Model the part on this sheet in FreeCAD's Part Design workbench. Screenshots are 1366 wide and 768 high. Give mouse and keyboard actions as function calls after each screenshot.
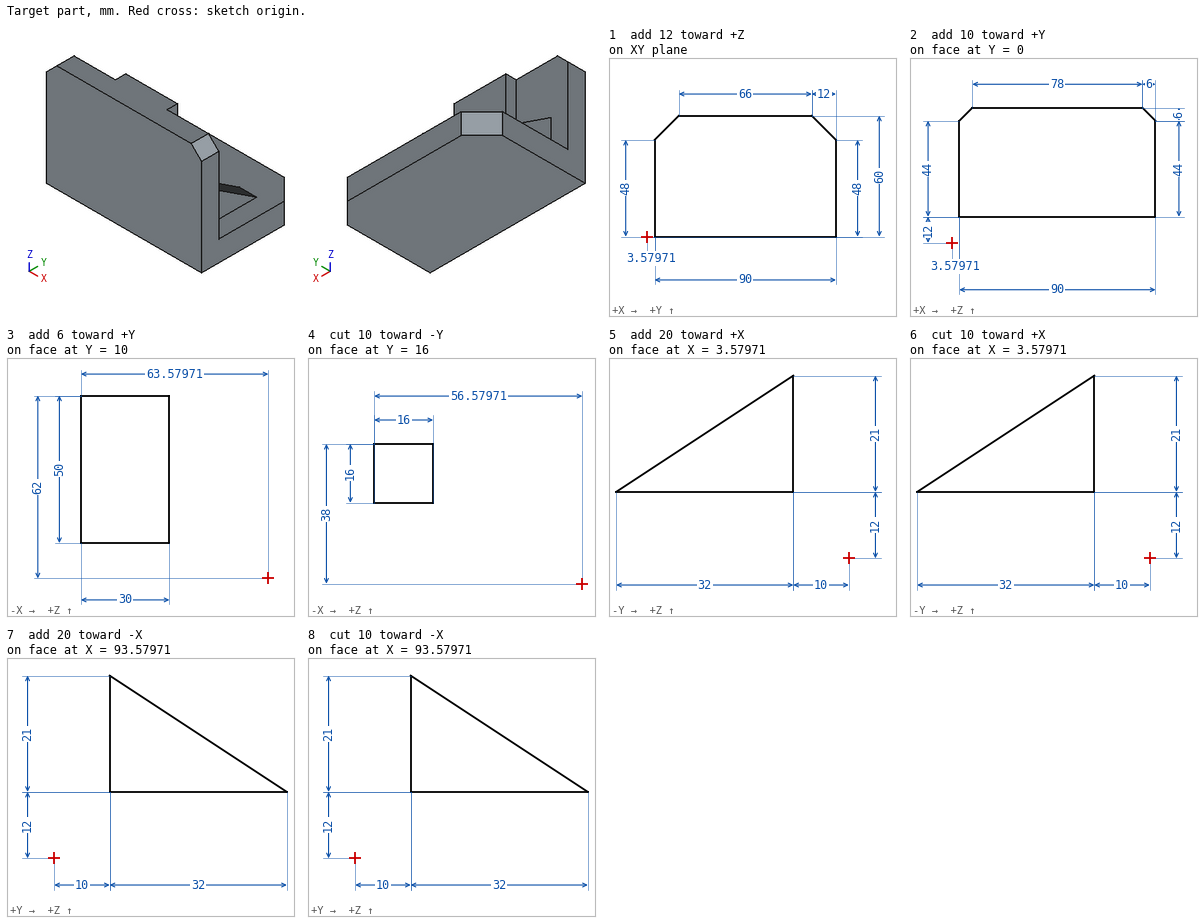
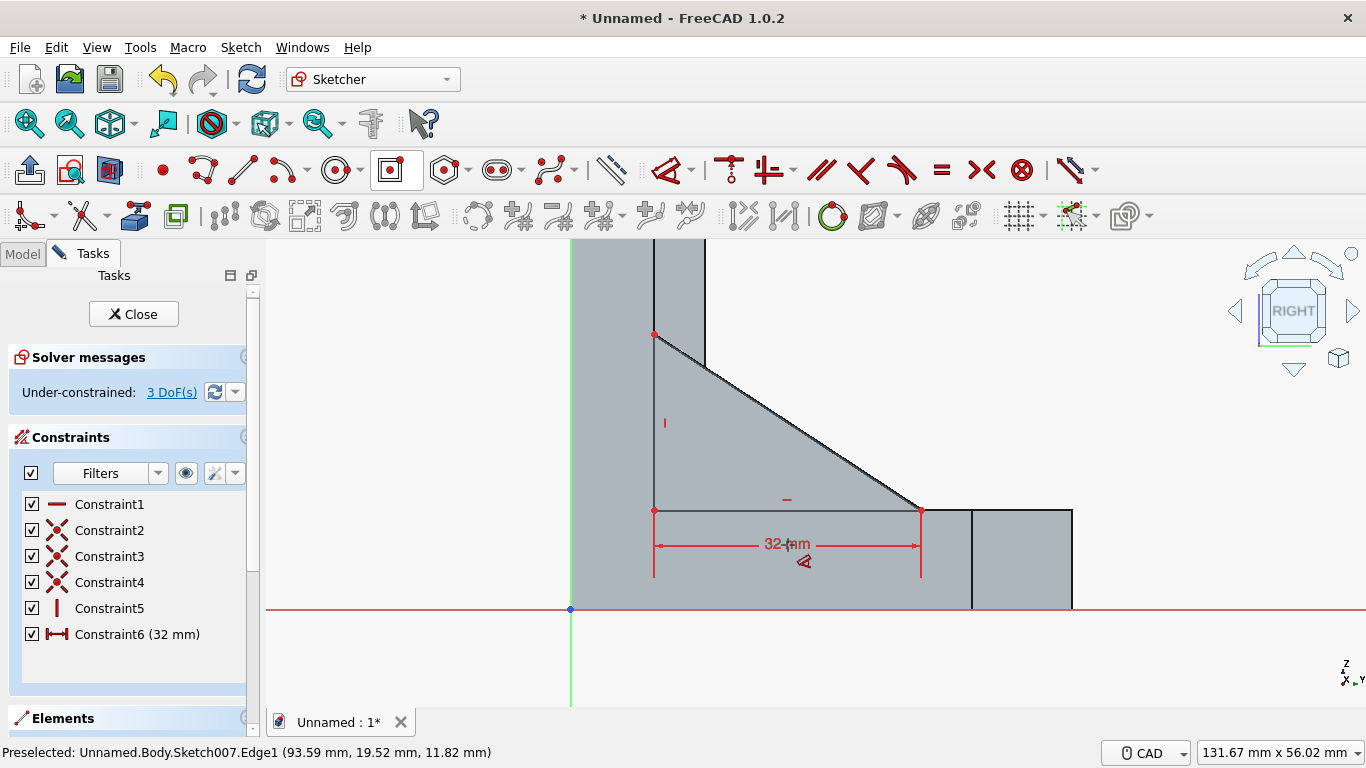
click(654, 388)
click(620, 423)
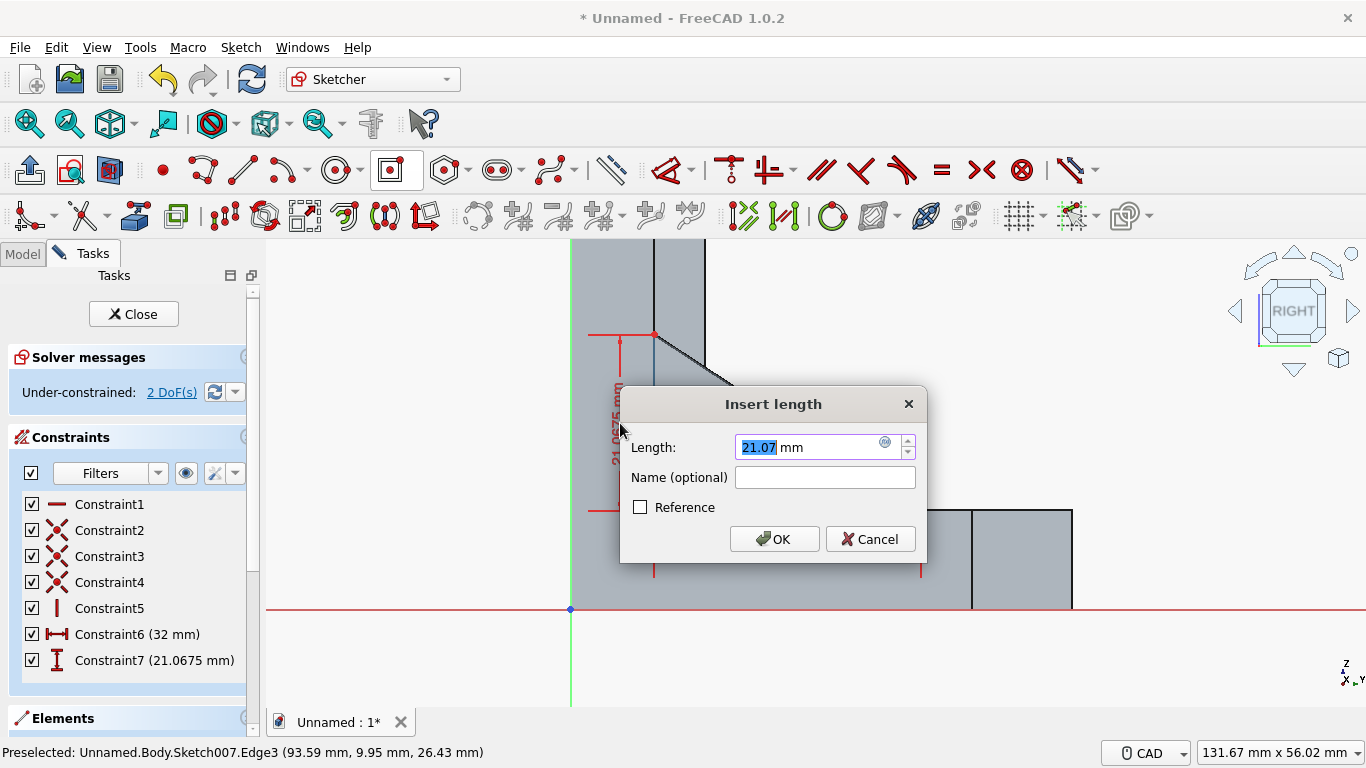
text(21)
key(Return)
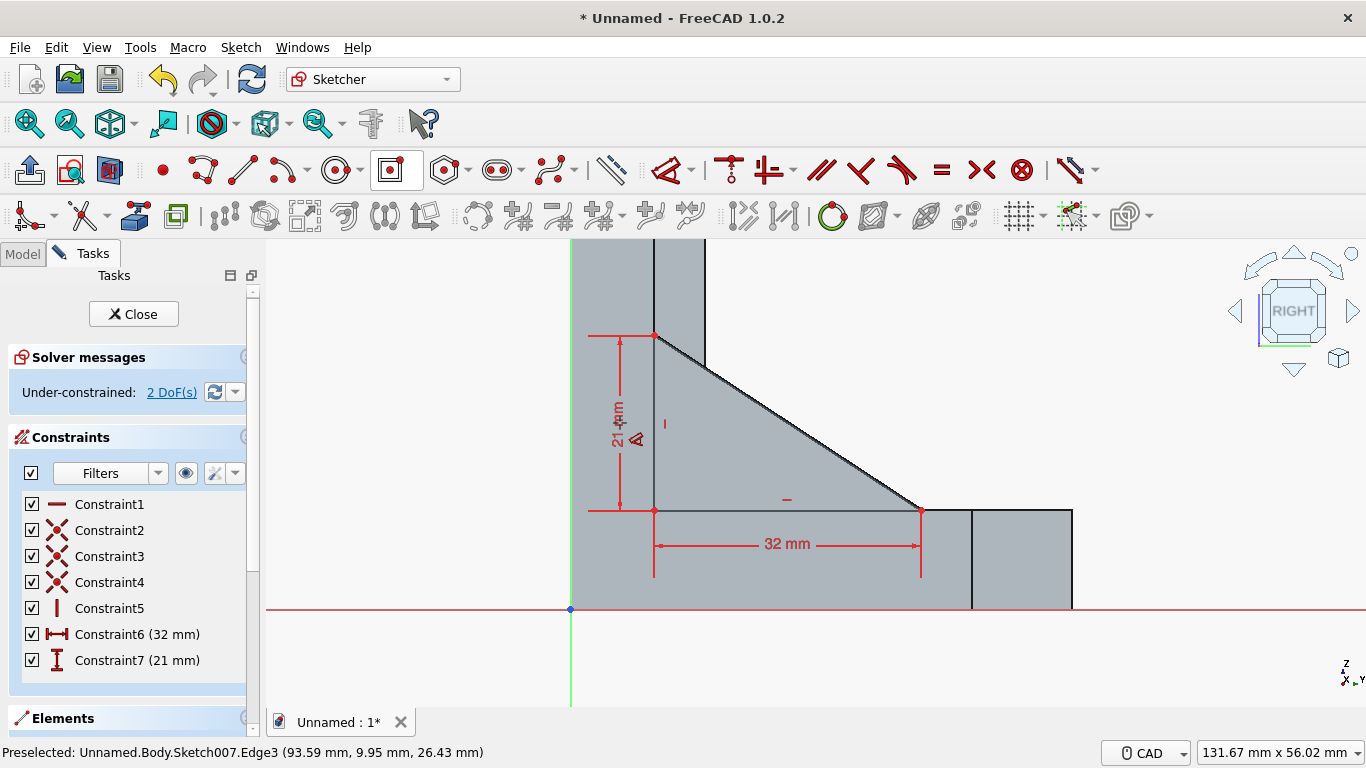
click(654, 511)
click(612, 644)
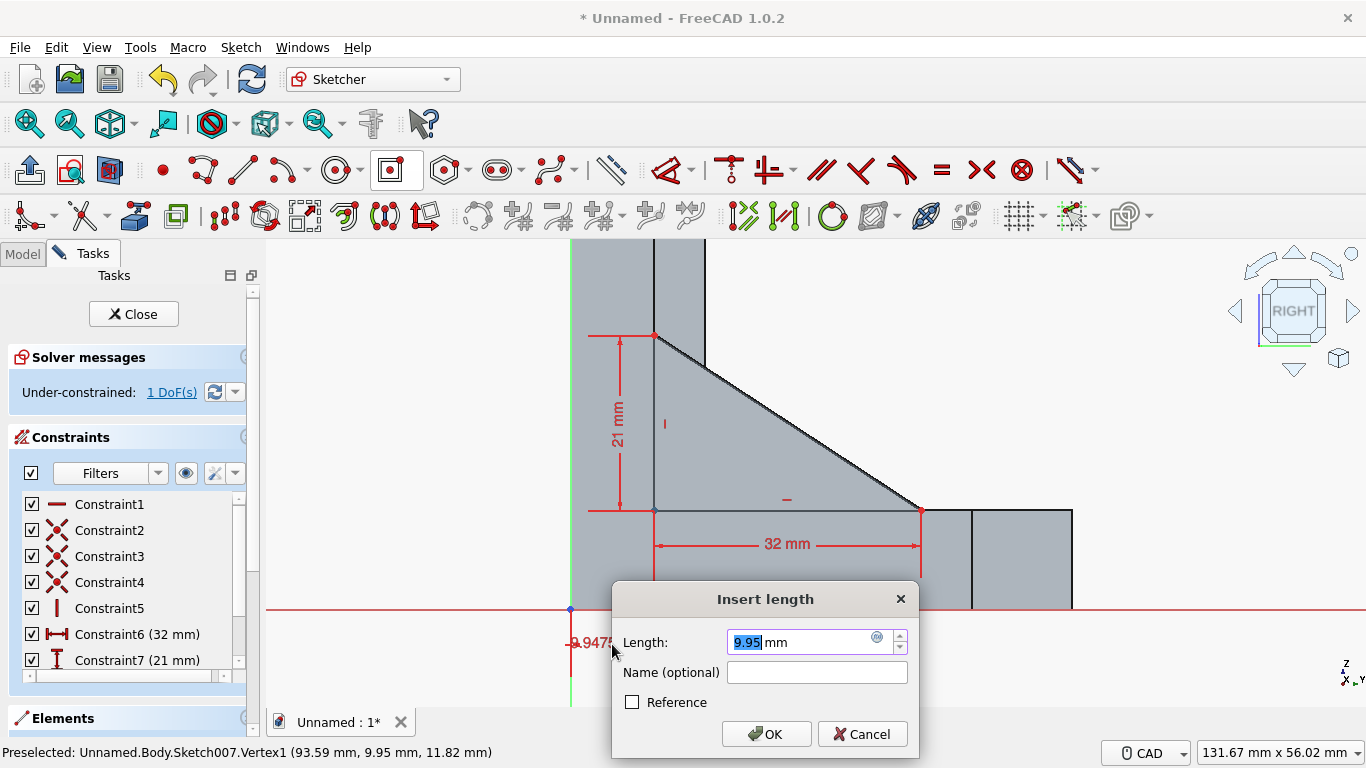
text(10)
key(Return)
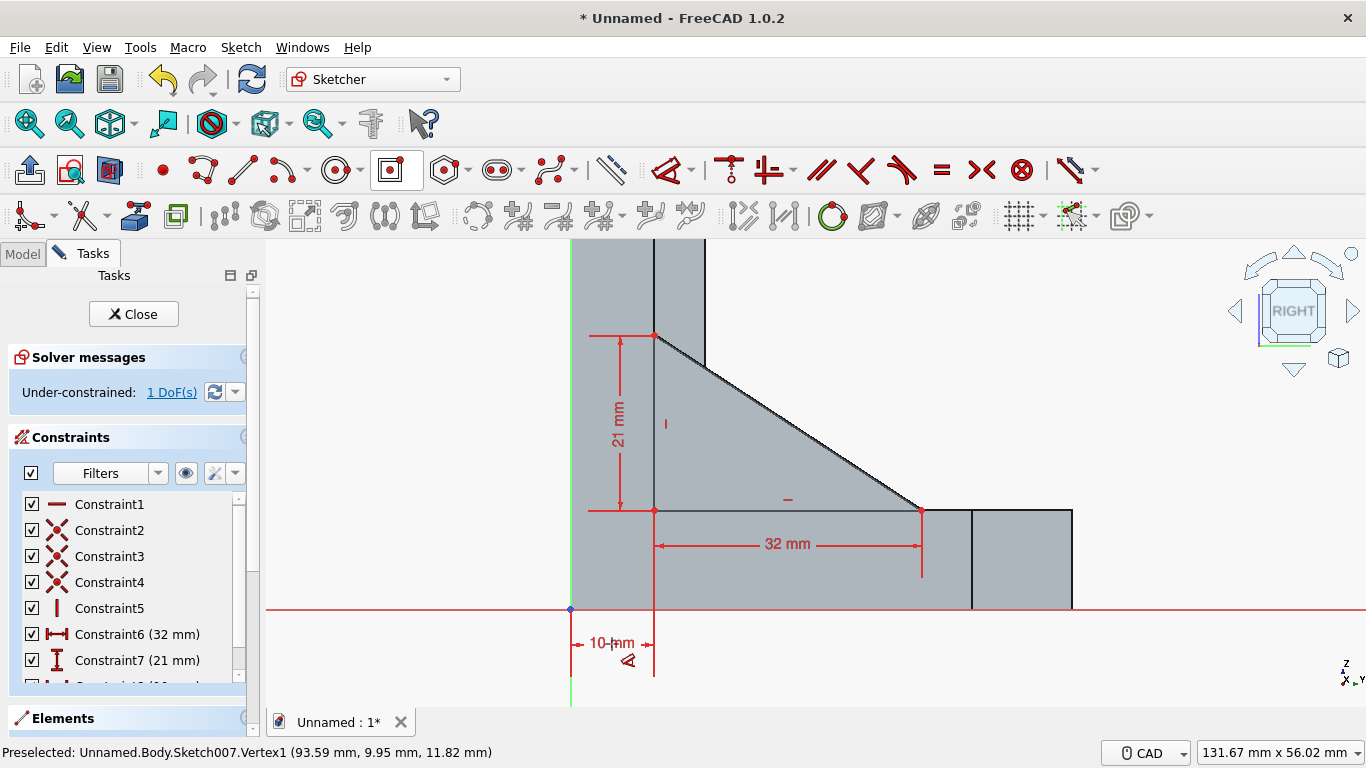
click(654, 511)
click(537, 560)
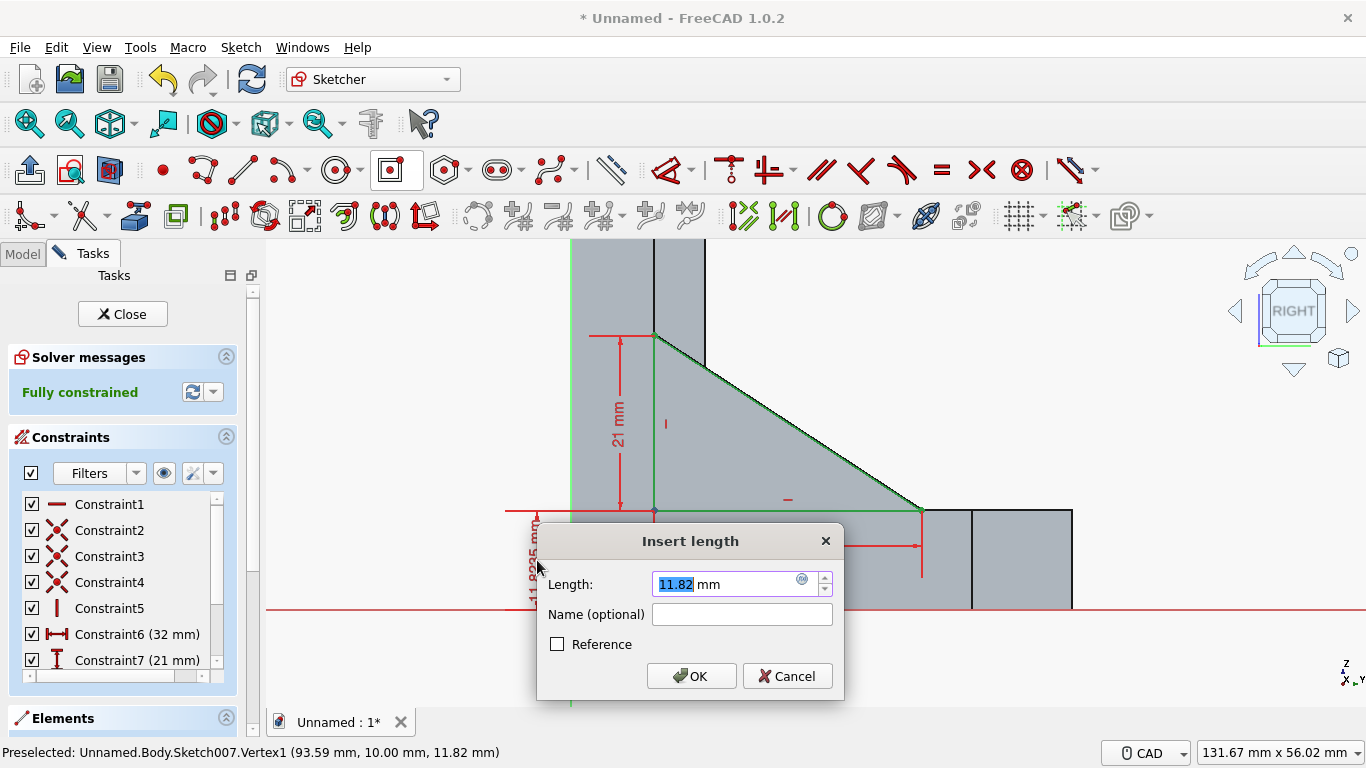
text(12)
key(Return)
key(Escape)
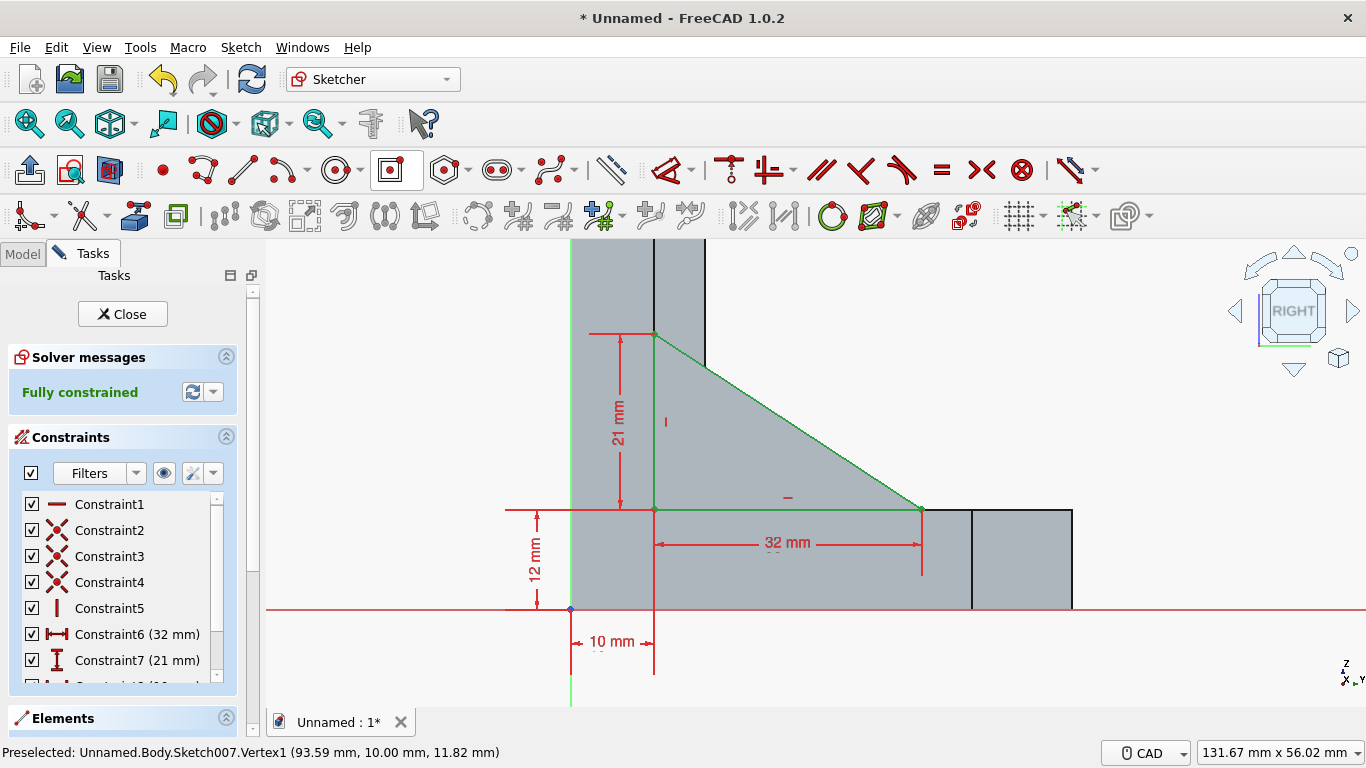
click(123, 314)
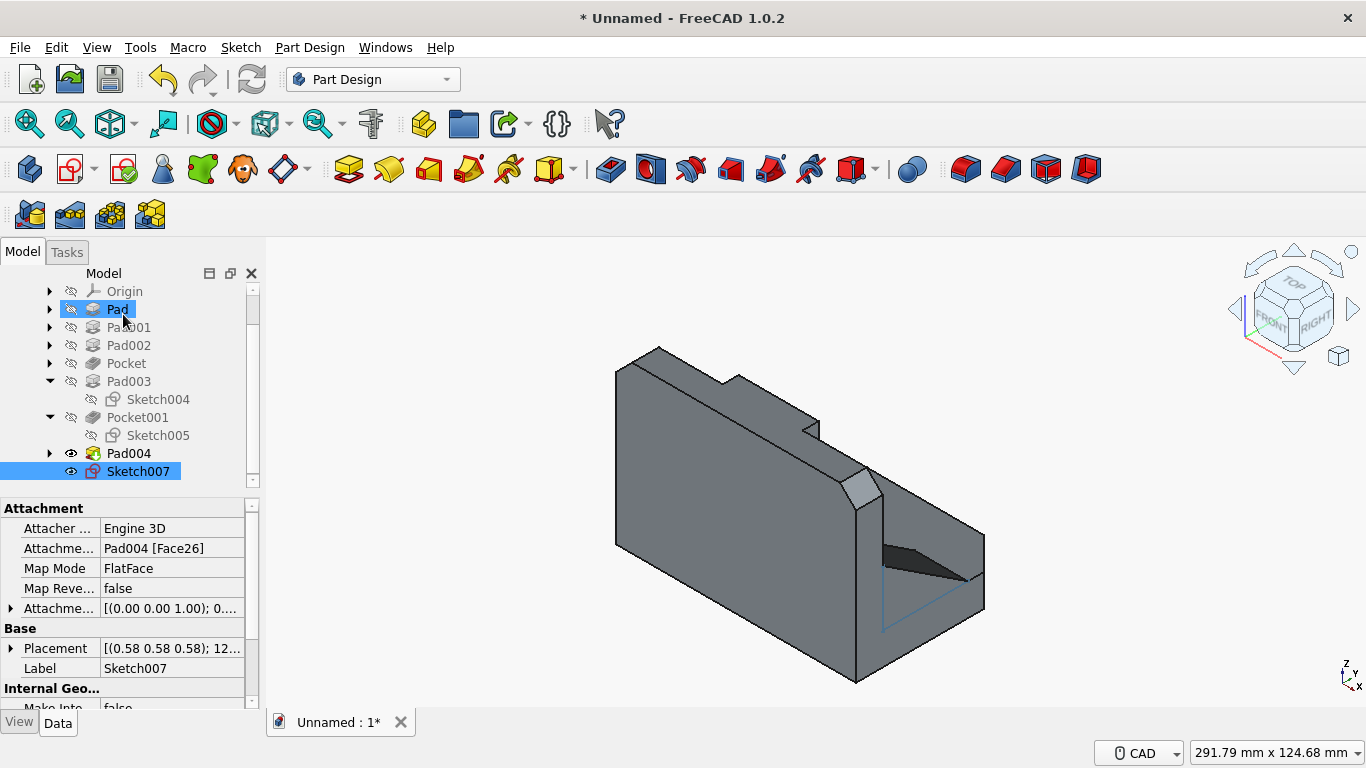
click(612, 170)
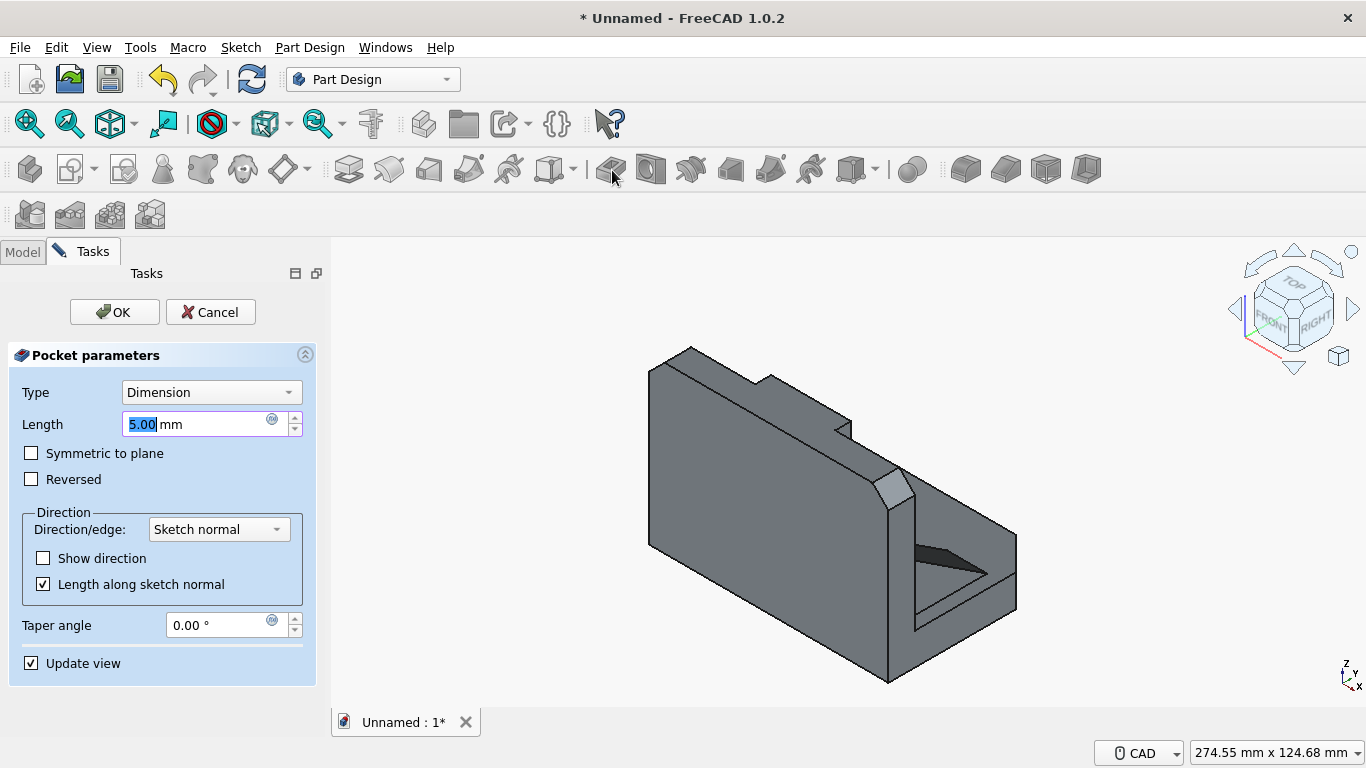
text(10)
key(Tab)